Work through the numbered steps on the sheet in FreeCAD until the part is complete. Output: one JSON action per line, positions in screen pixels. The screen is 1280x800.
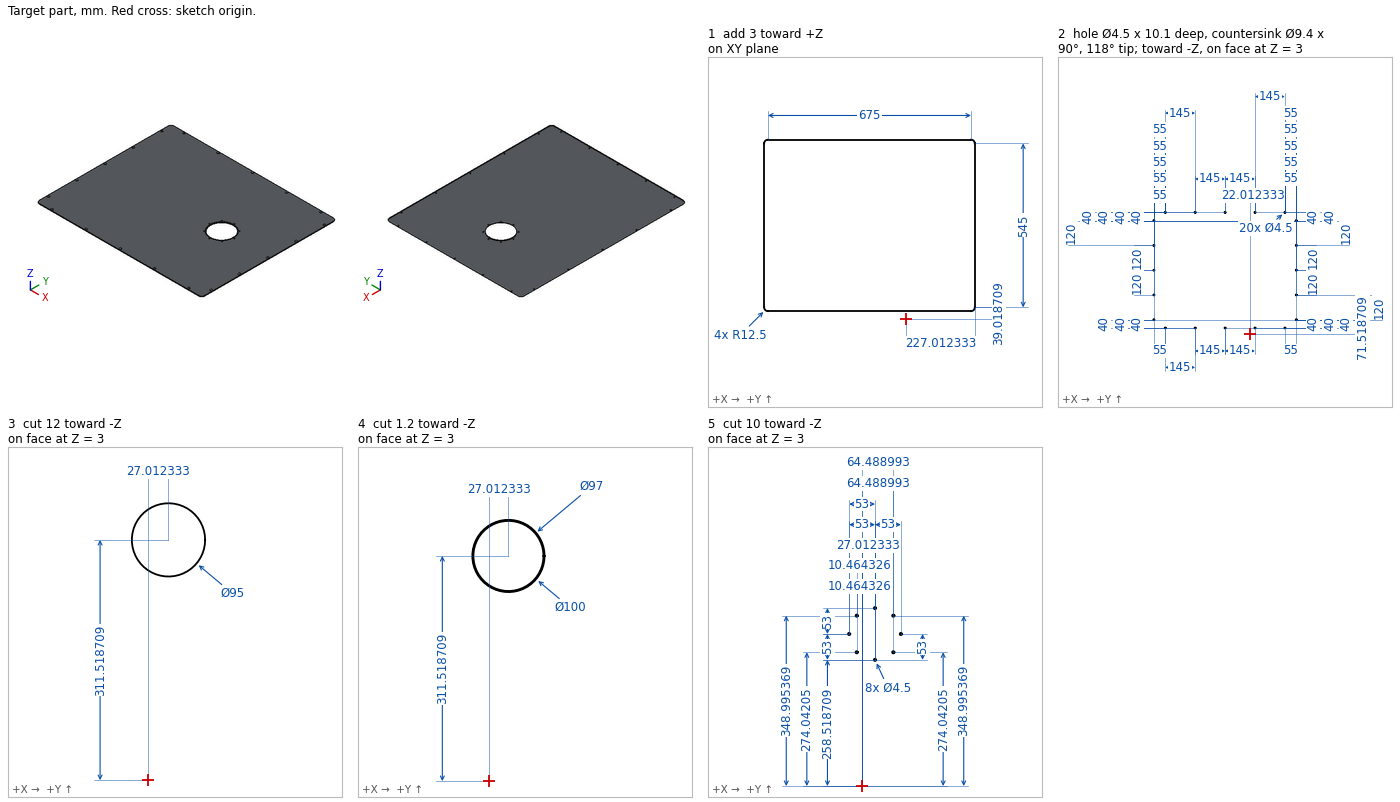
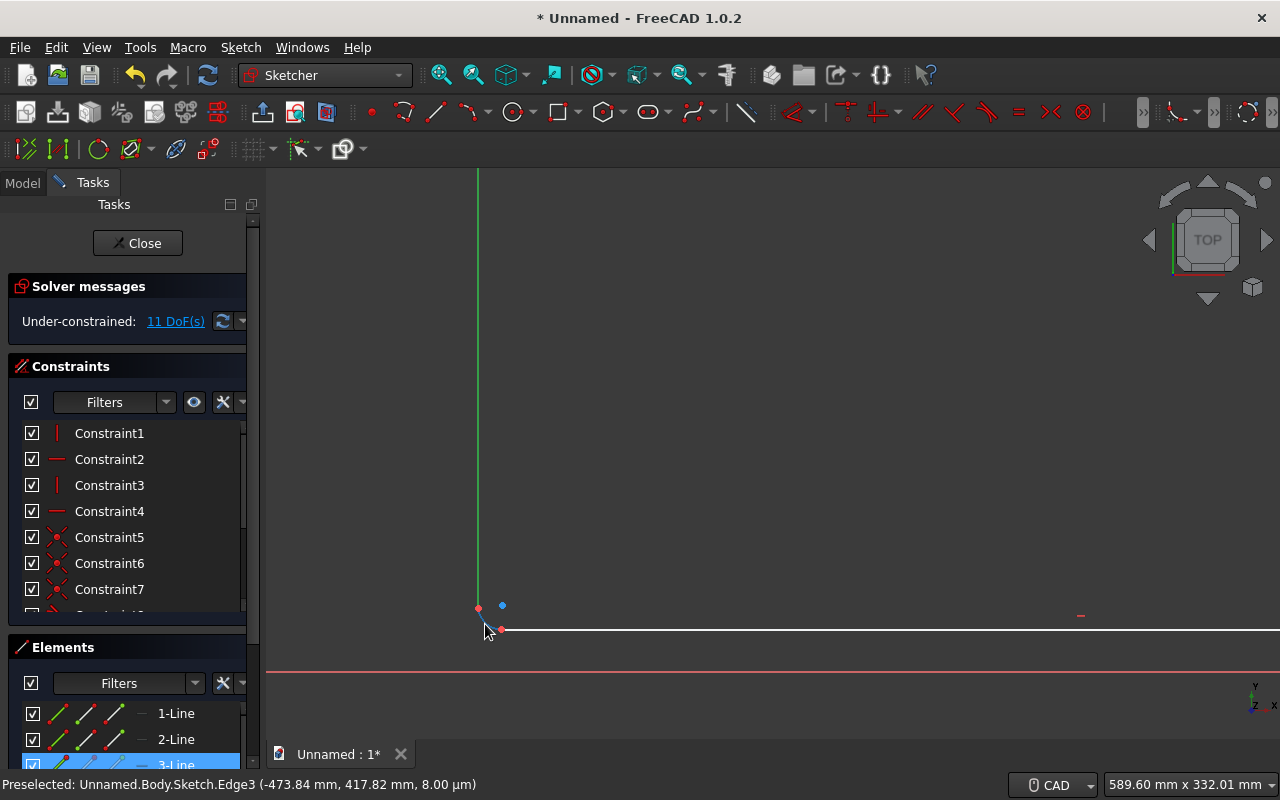
{"action": "left_click", "coordinate": [486, 623]}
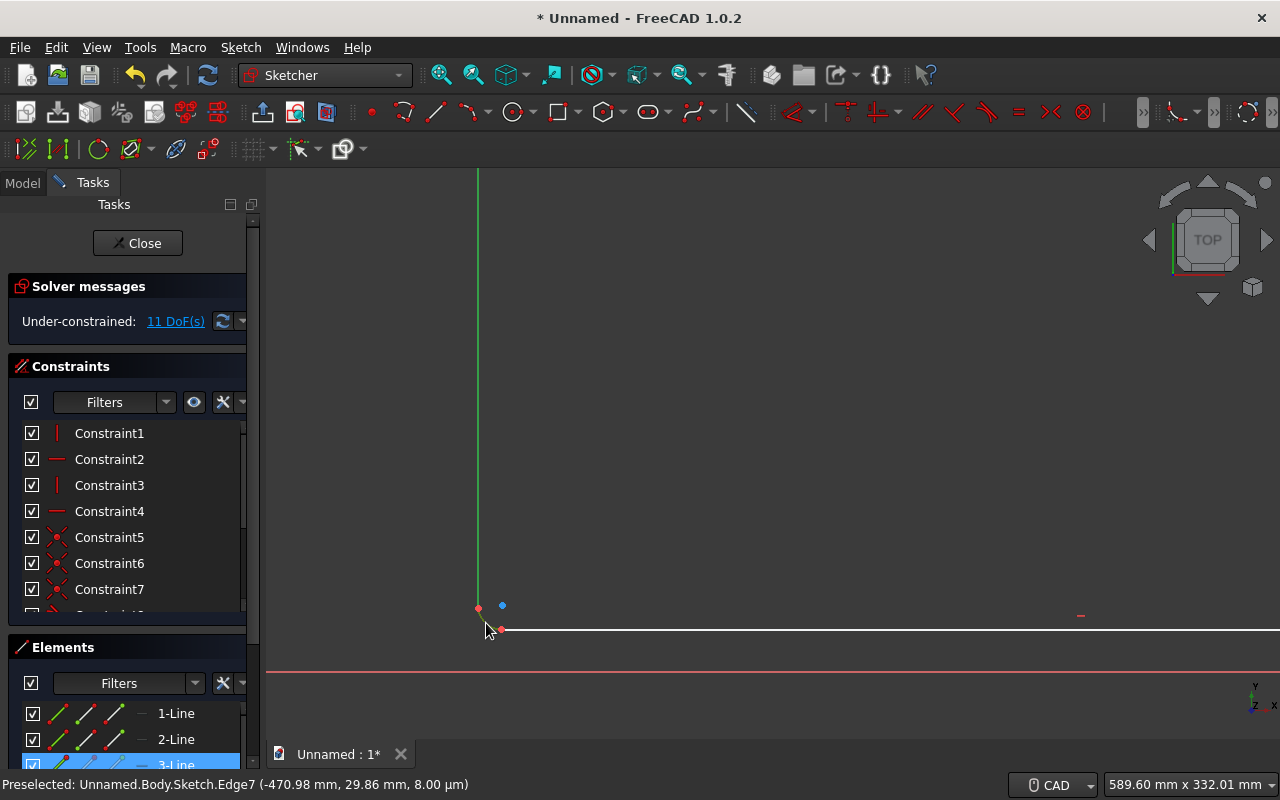
{"action": "left_click", "coordinate": [988, 112]}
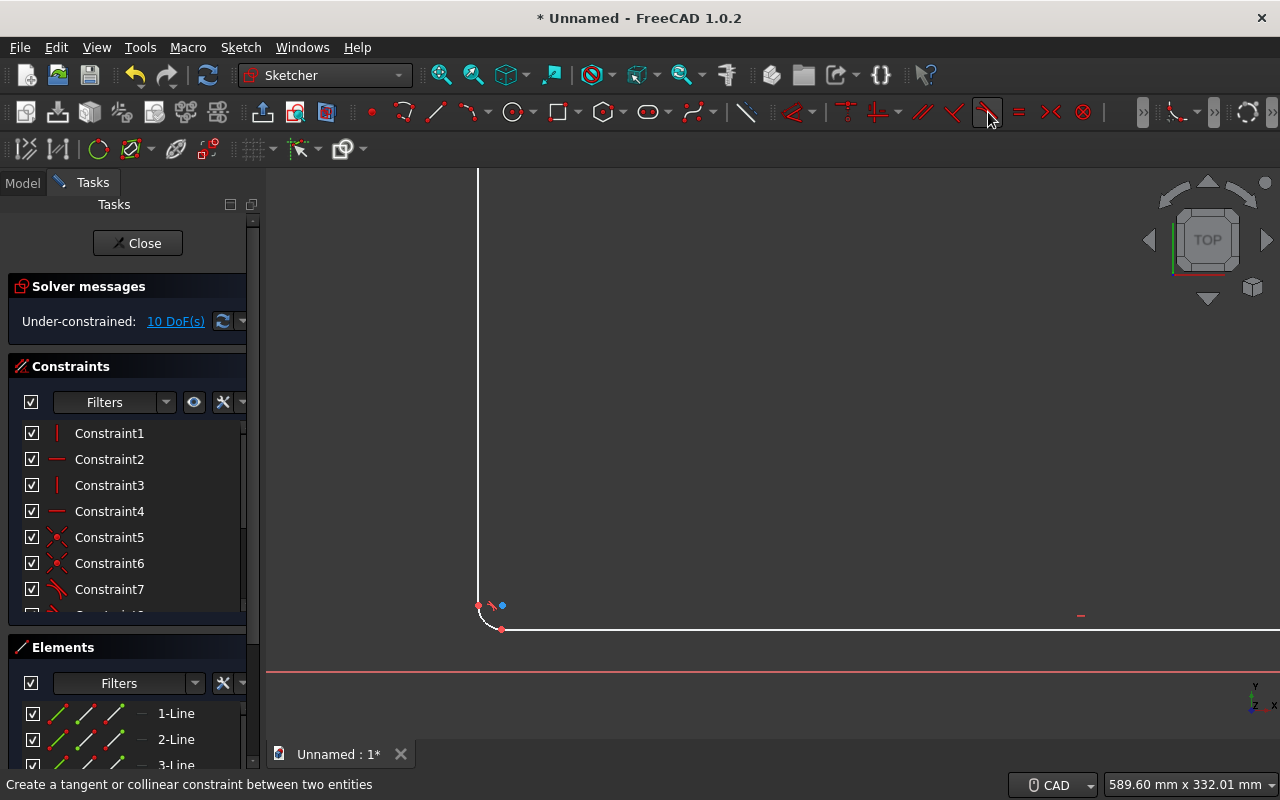
{"action": "left_click", "coordinate": [850, 630]}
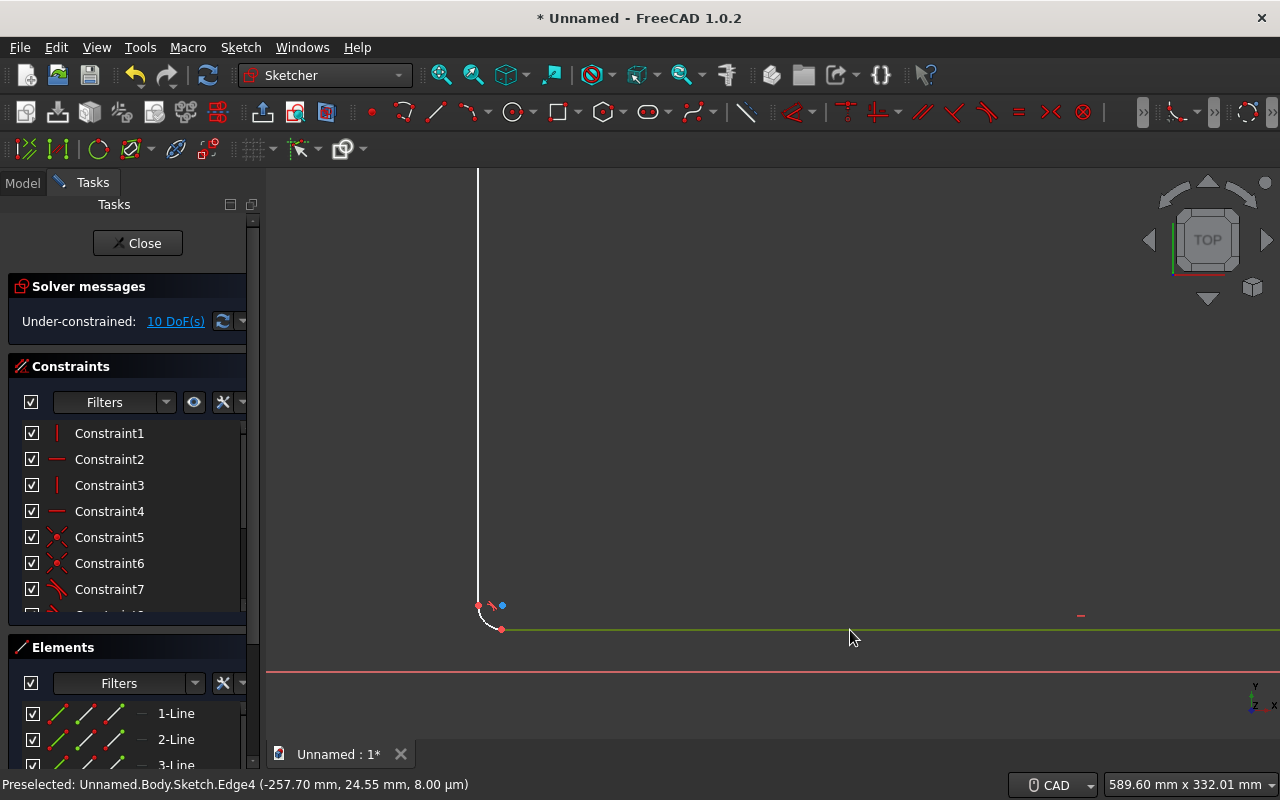
{"action": "scroll", "coordinate": [481, 616], "scroll_direction": "up", "scroll_amount": 2}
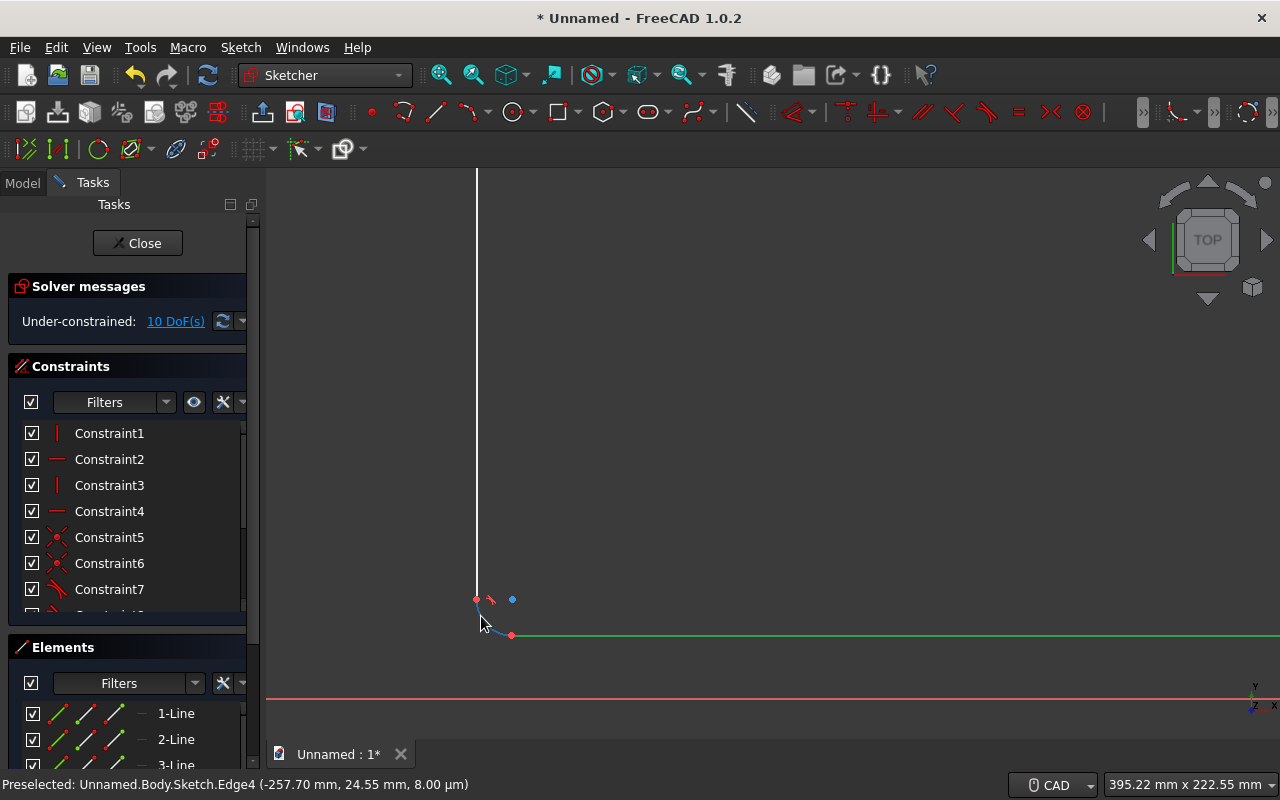
{"action": "left_click", "coordinate": [481, 616]}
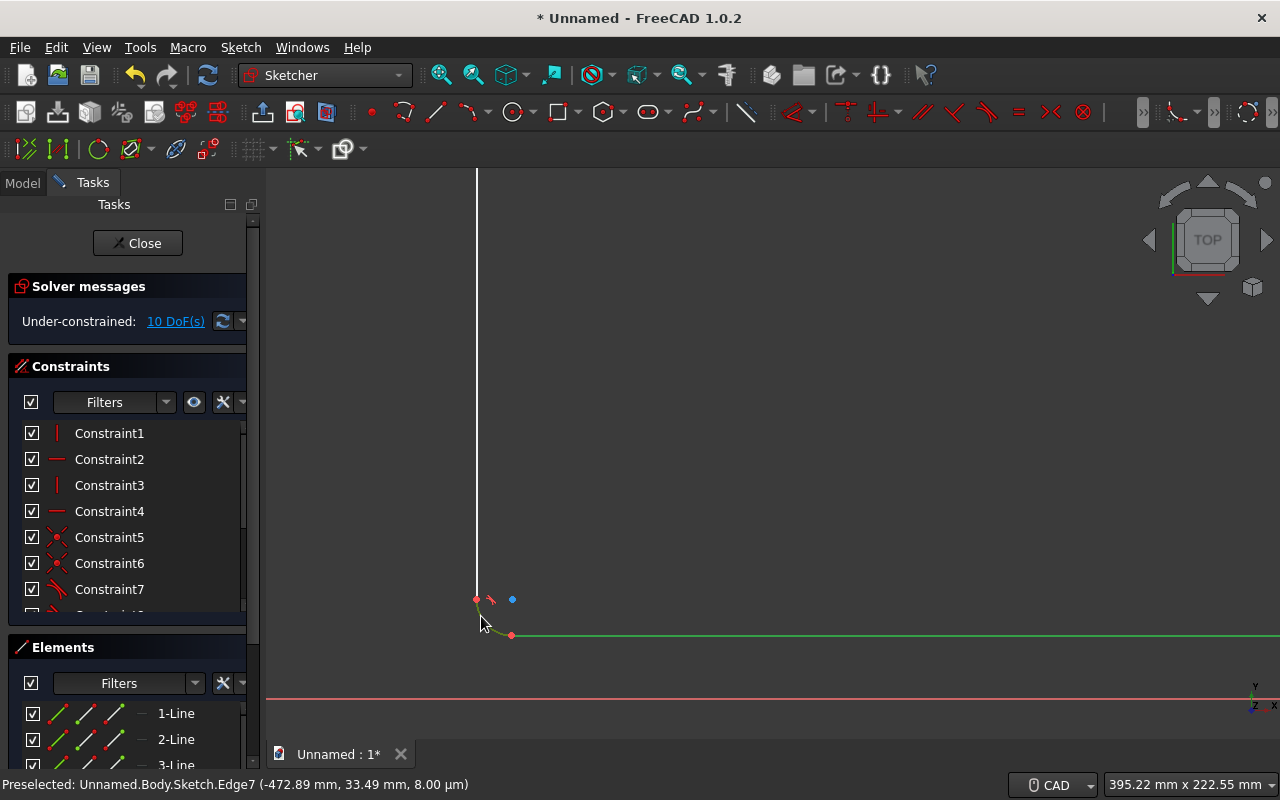
{"action": "left_click", "coordinate": [988, 112]}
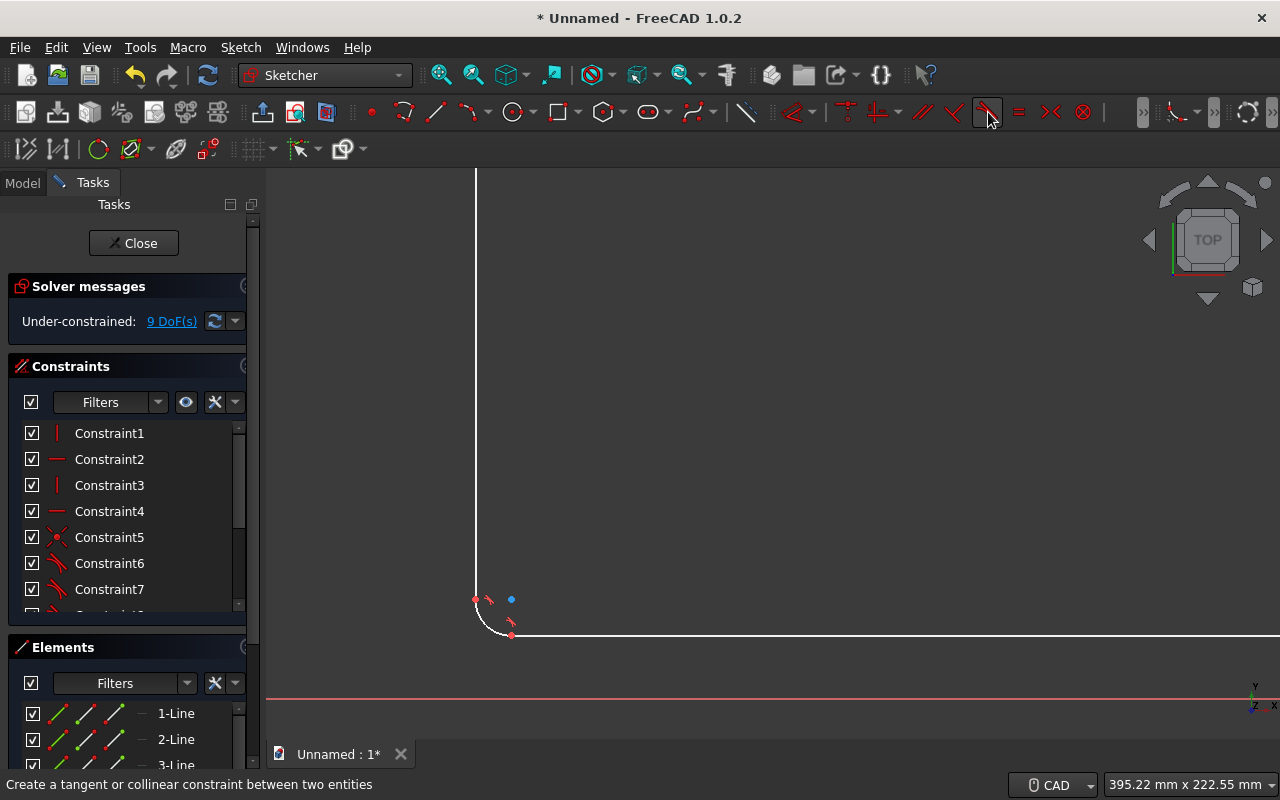
{"action": "scroll", "coordinate": [484, 624], "scroll_direction": "down", "scroll_amount": 7}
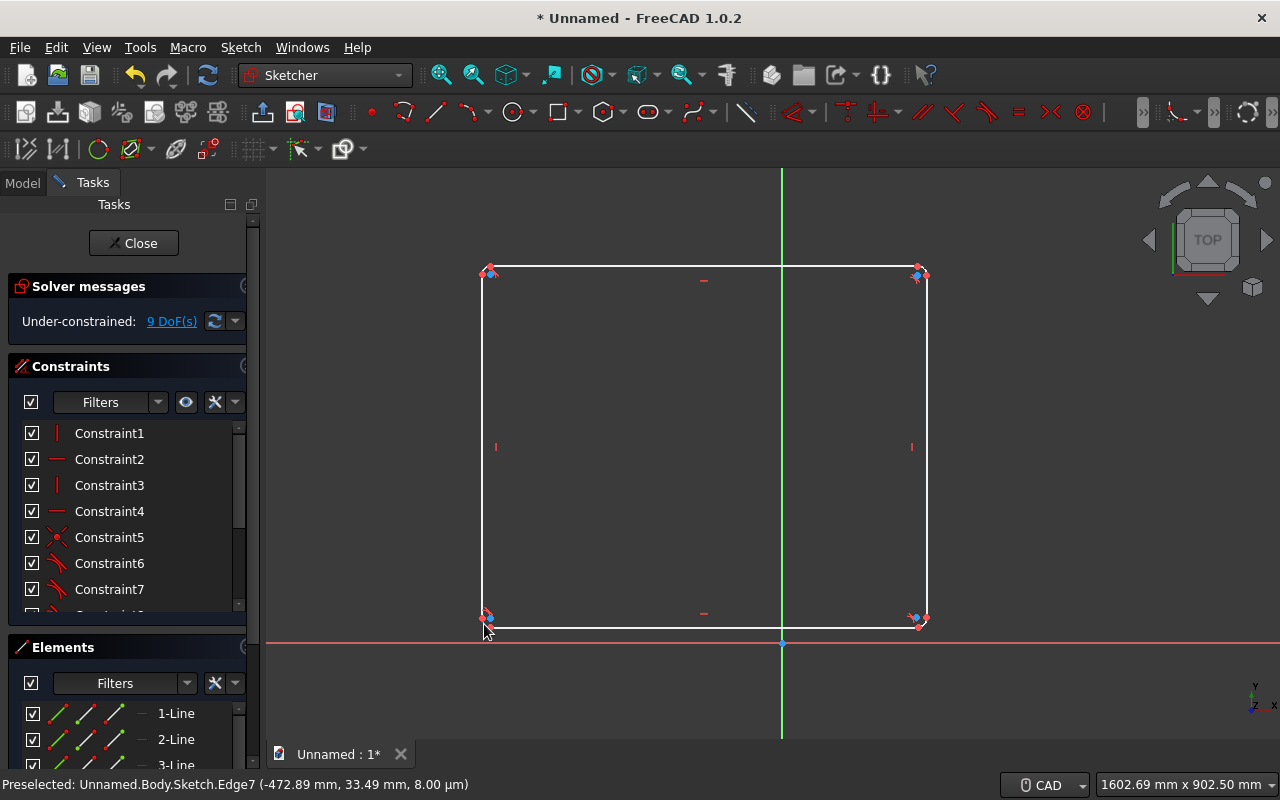
{"action": "left_click", "coordinate": [619, 628]}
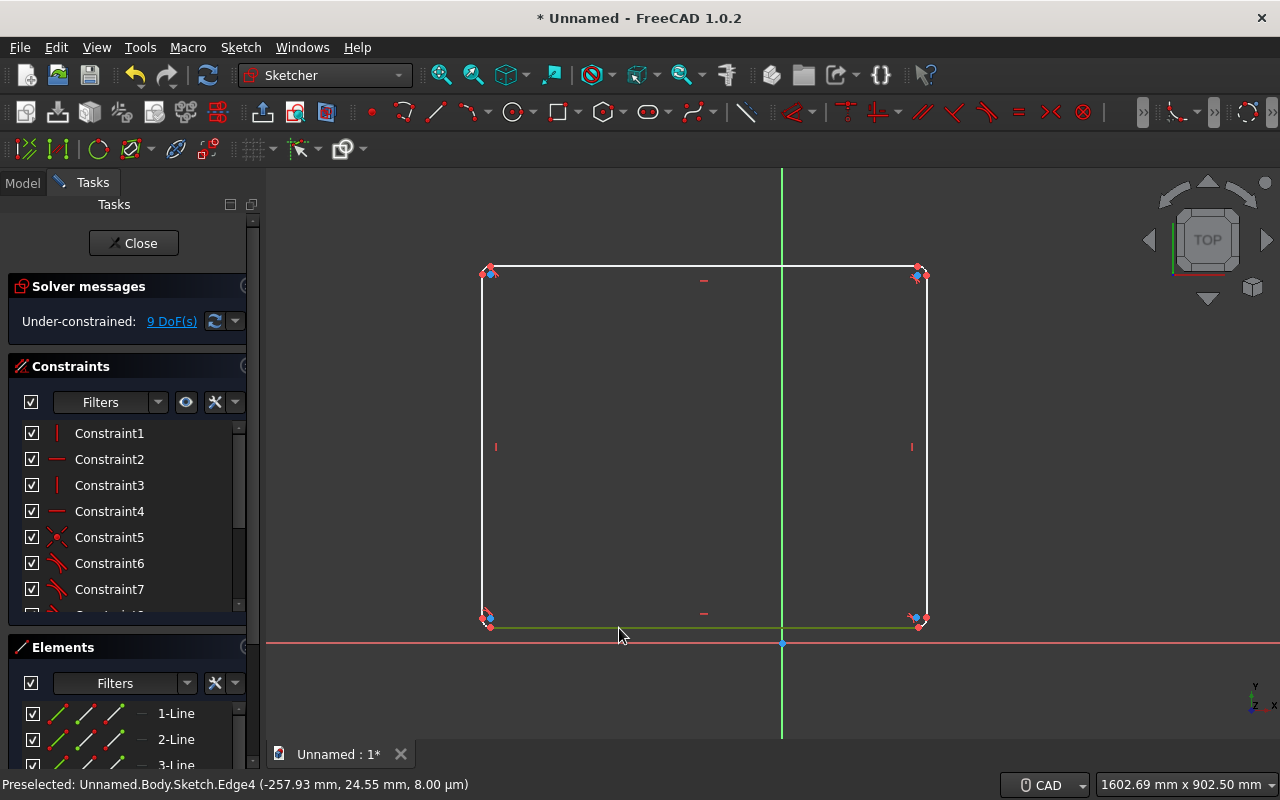
{"action": "scroll", "coordinate": [924, 624], "scroll_direction": "up", "scroll_amount": 4}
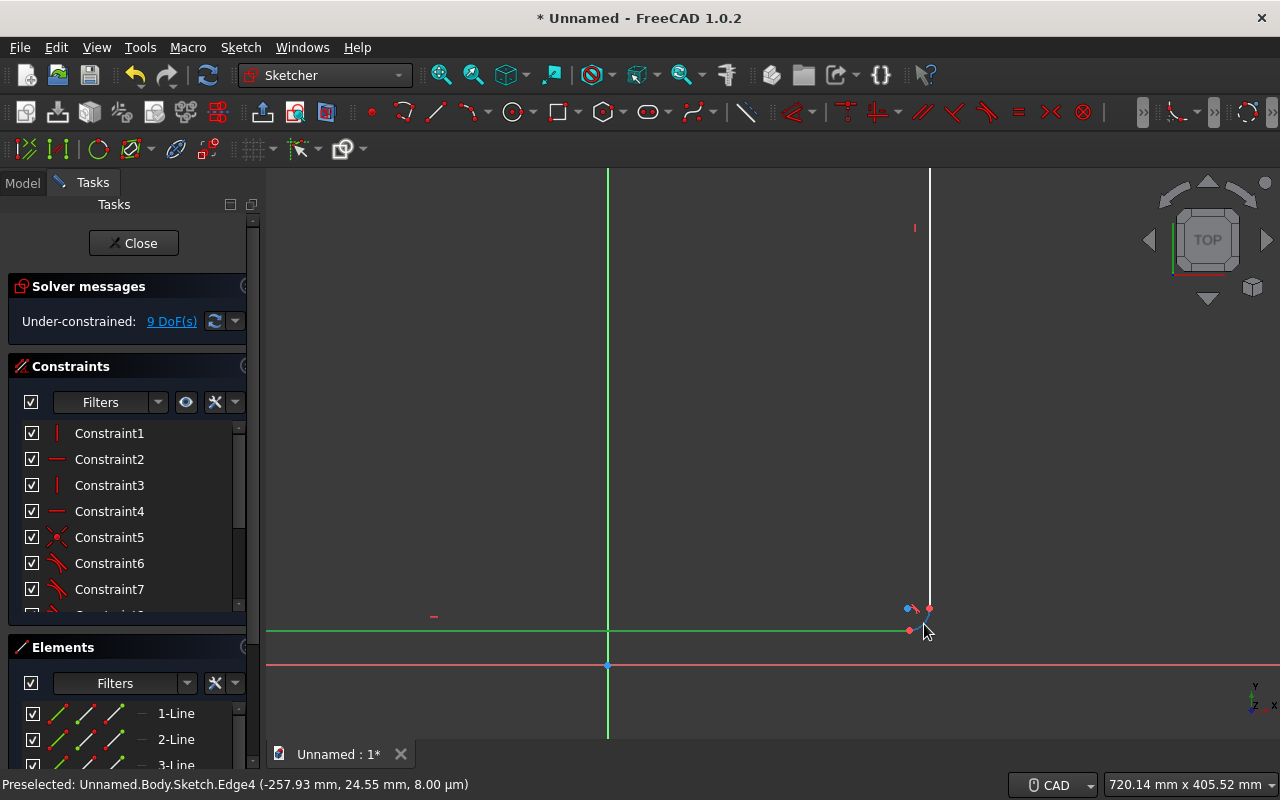
{"action": "left_click", "coordinate": [924, 623]}